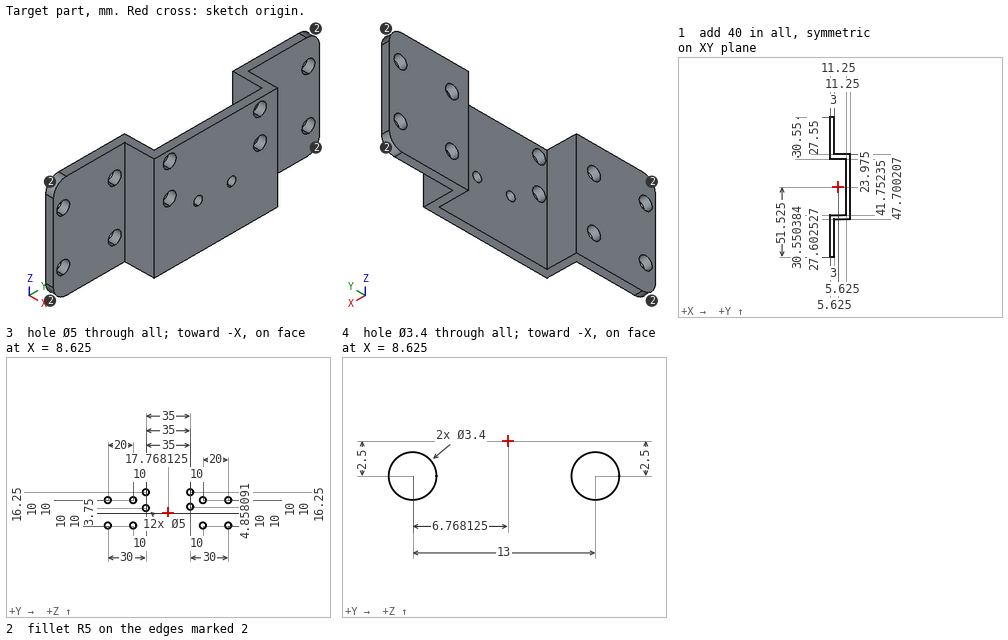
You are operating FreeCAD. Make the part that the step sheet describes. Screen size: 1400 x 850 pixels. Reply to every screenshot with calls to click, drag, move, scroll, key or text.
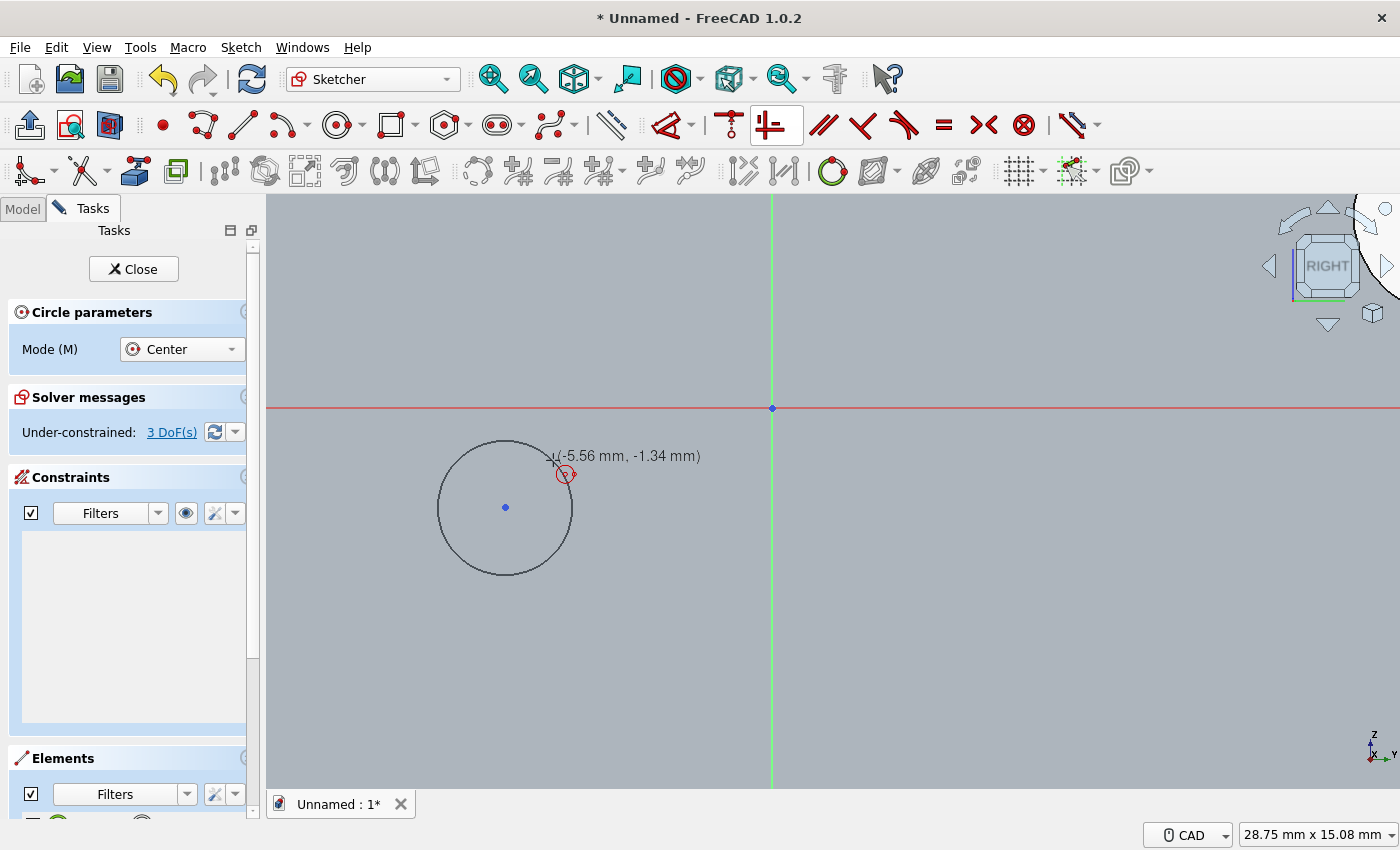
click(1018, 507)
click(1065, 460)
key(Escape)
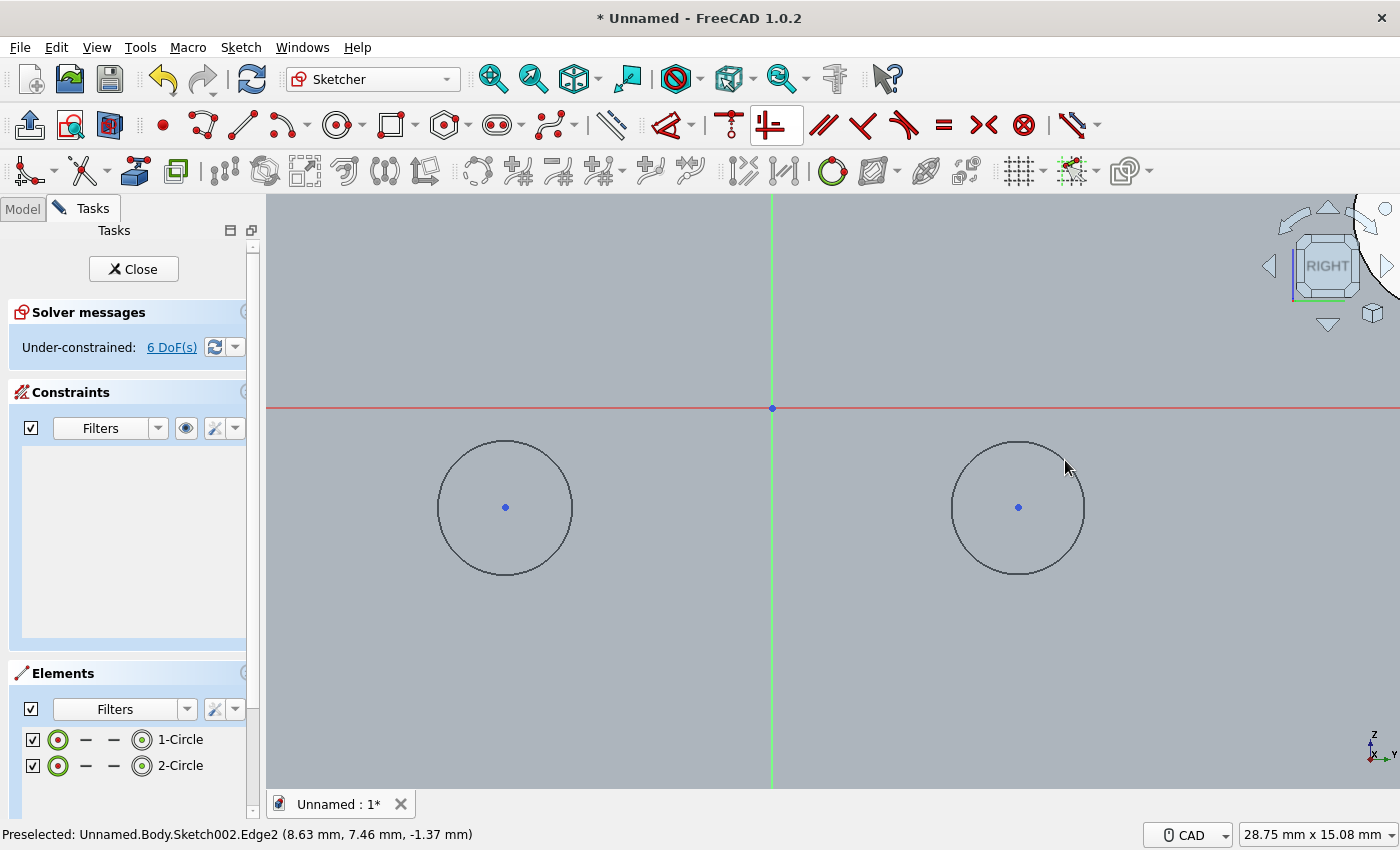
click(552, 460)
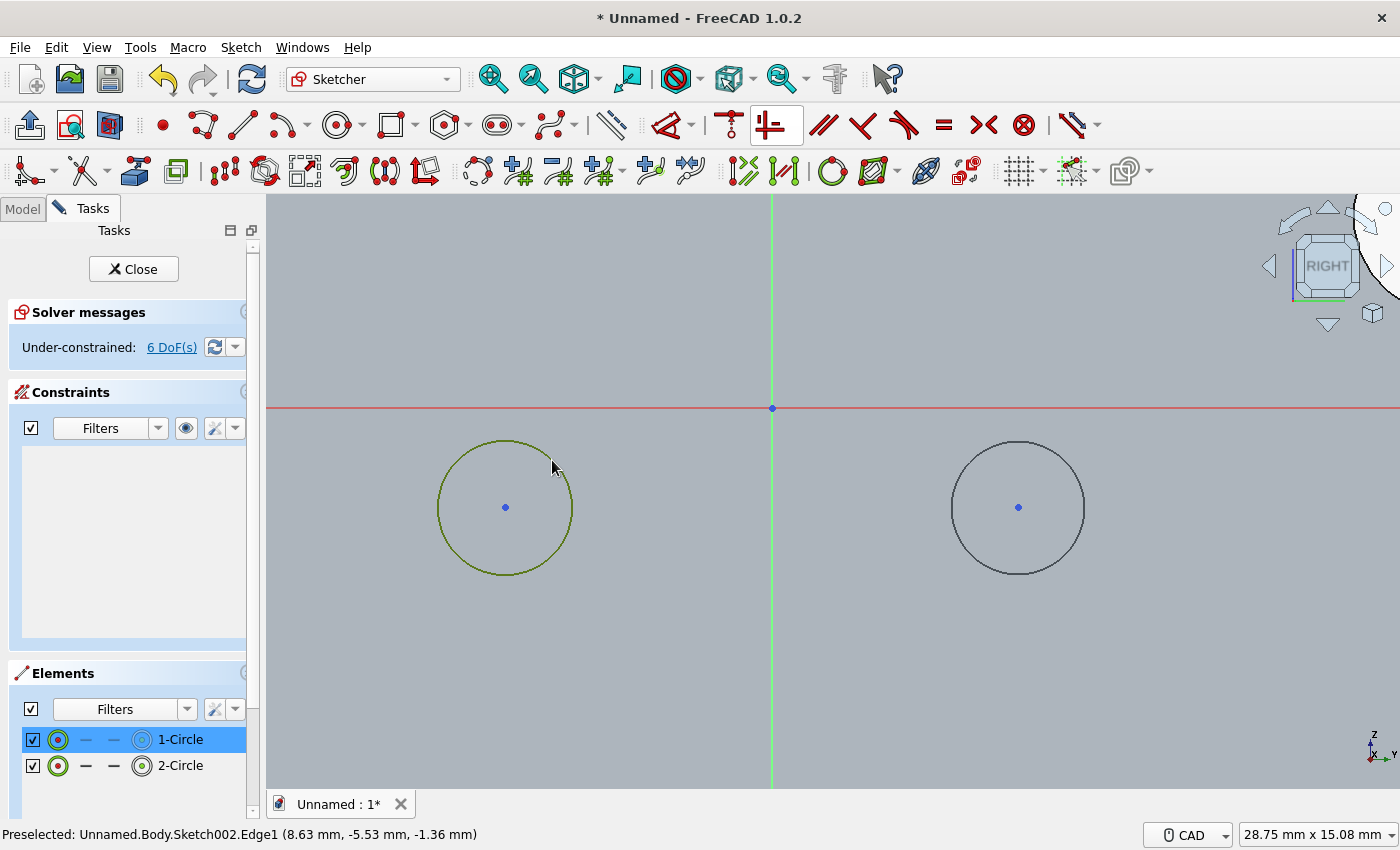
click(1065, 461)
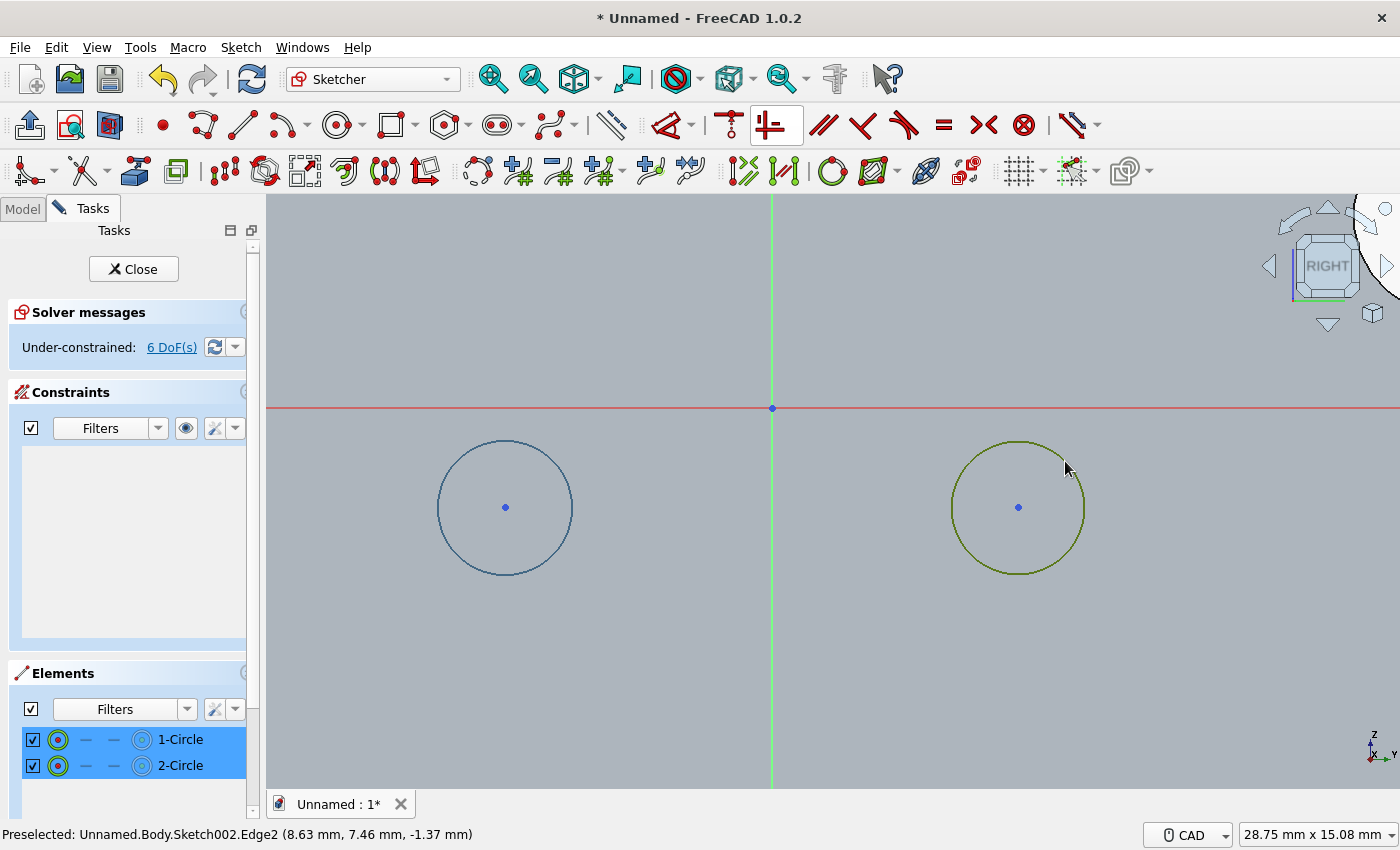
click(944, 126)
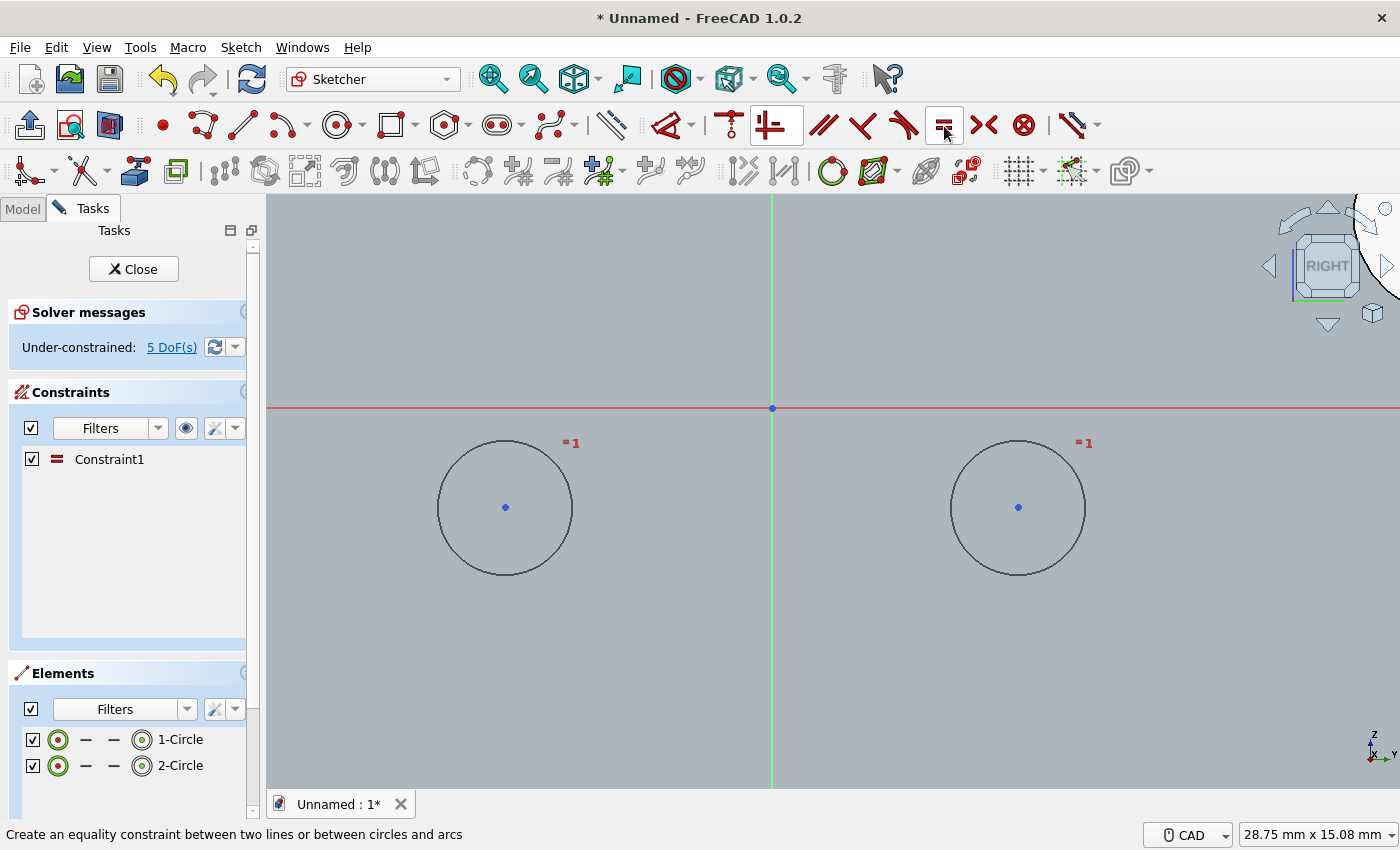
key(d)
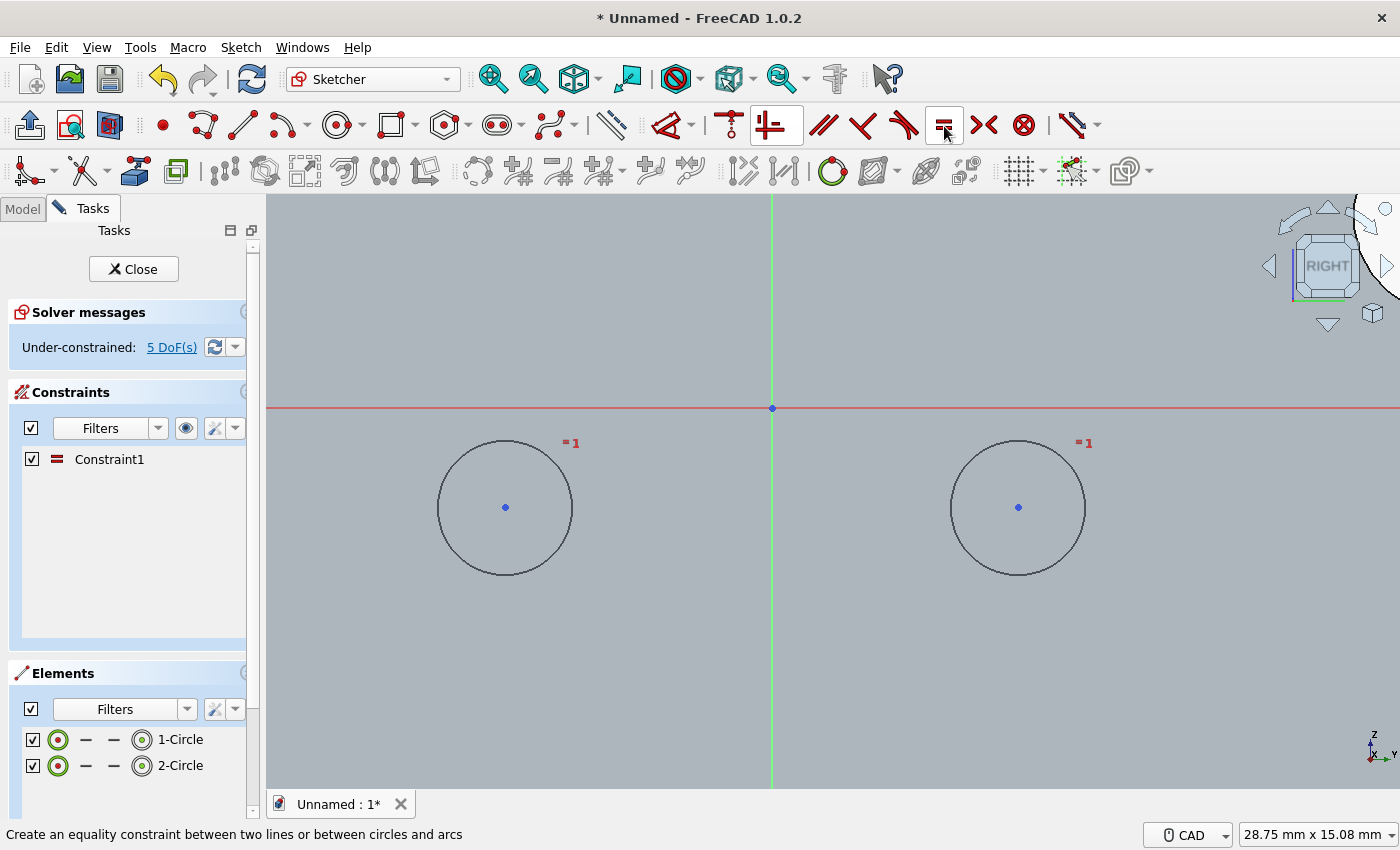
click(552, 460)
click(574, 437)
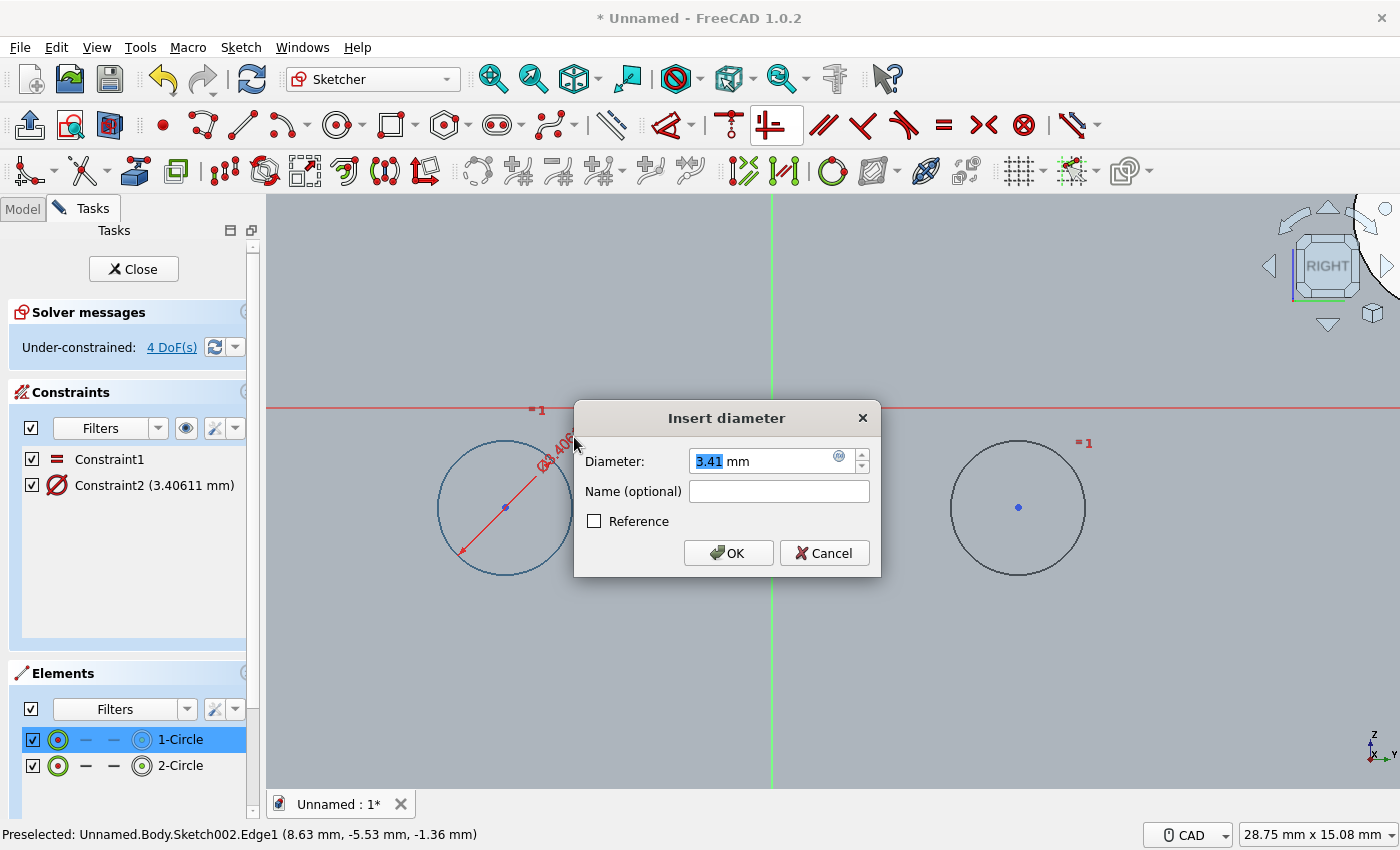
text(3.4)
key(Return)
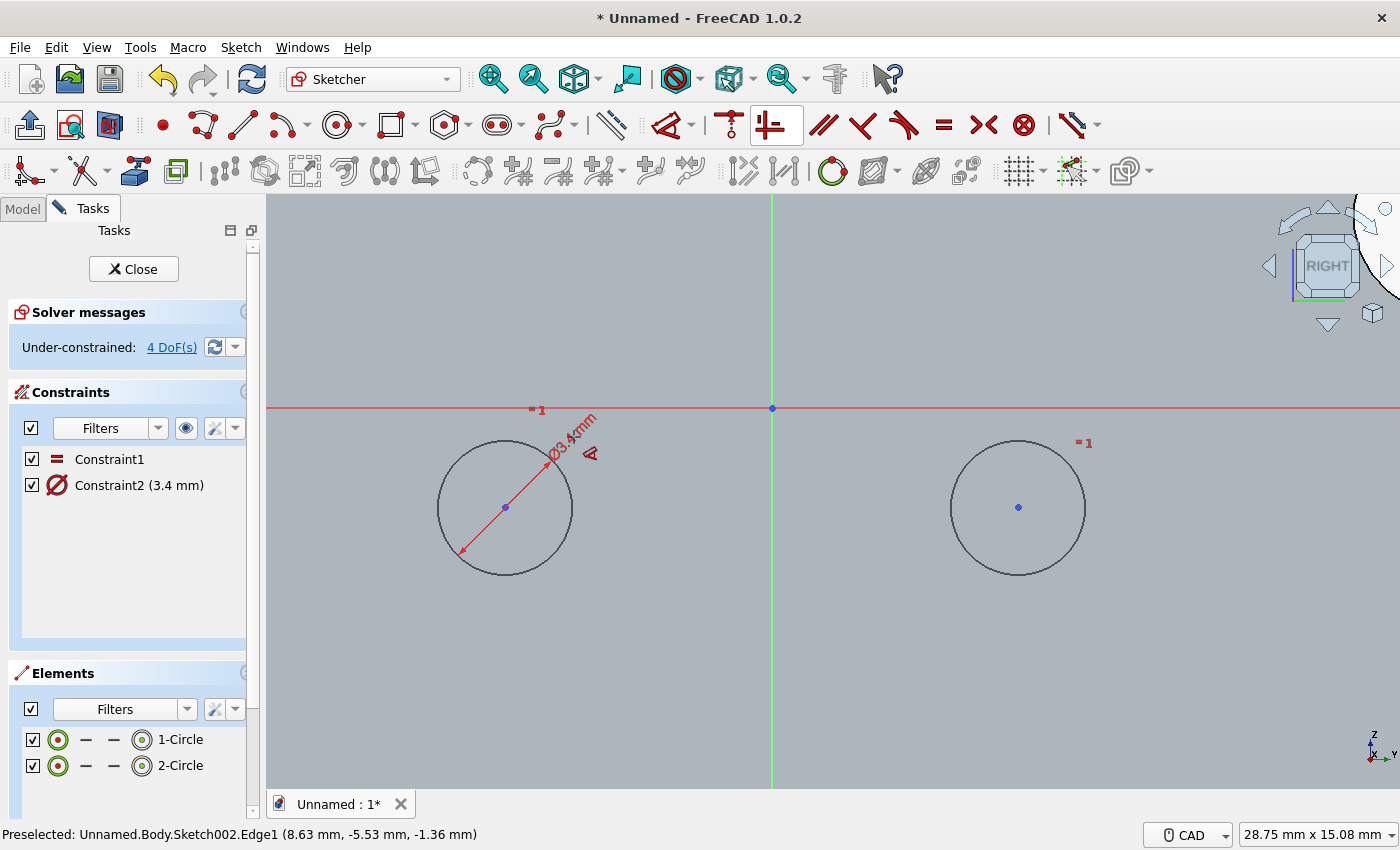
click(505, 508)
click(471, 435)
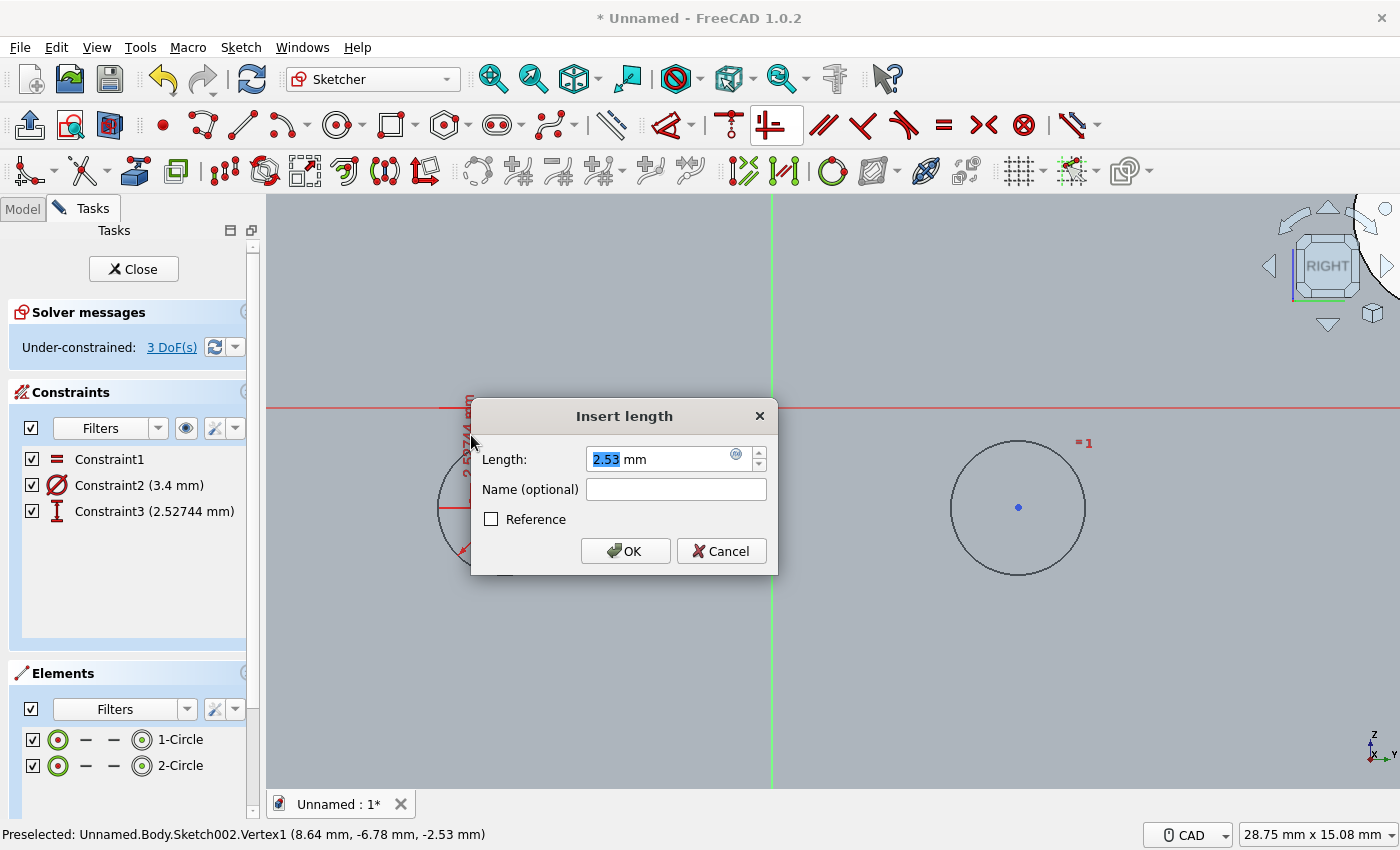
text(2.5)
key(Return)